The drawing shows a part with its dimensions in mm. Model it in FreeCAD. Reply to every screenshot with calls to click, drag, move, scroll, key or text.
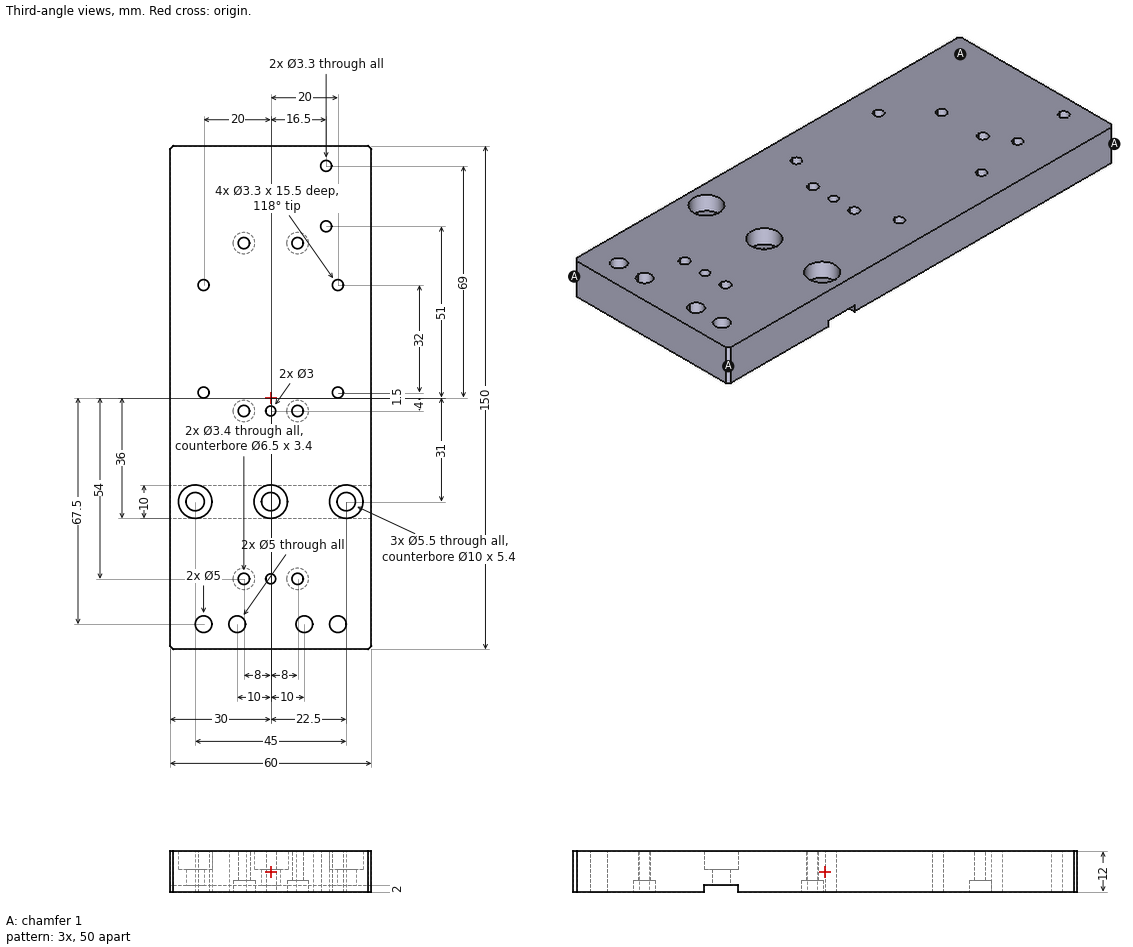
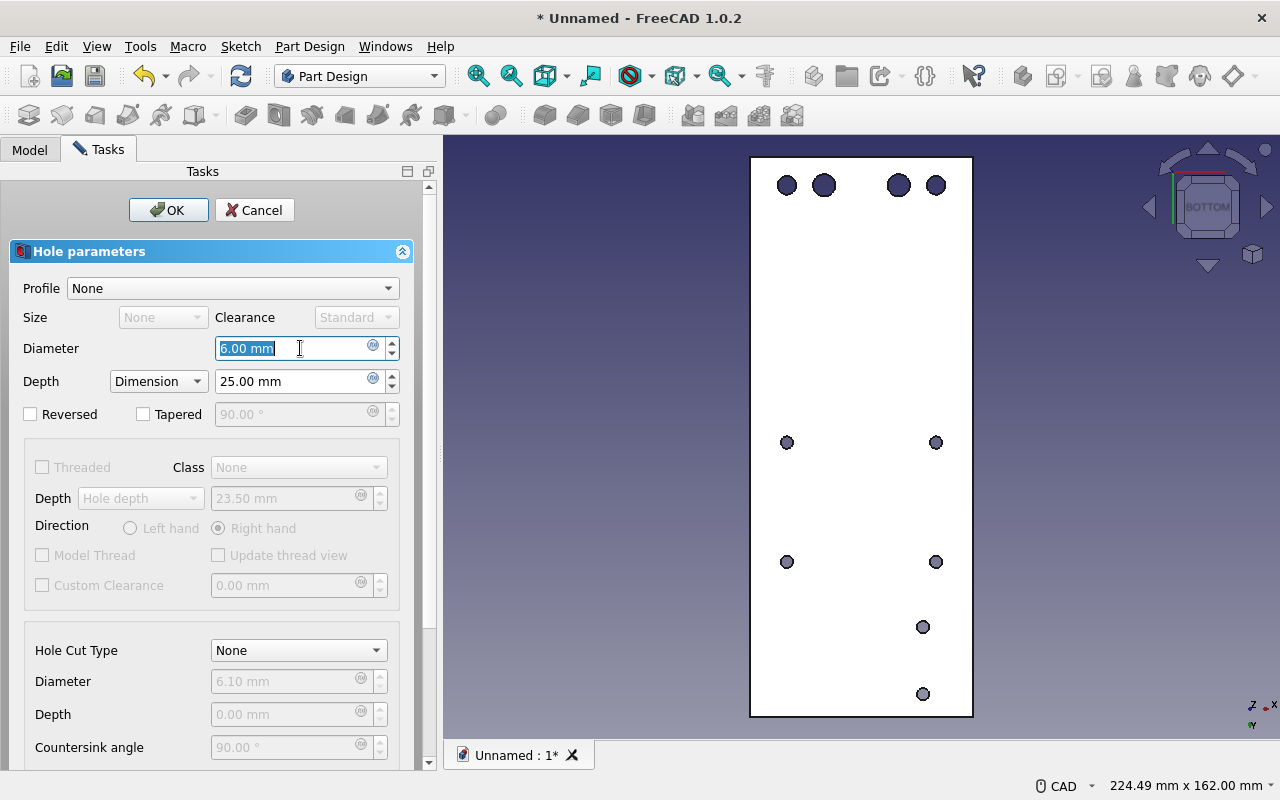
text(5)
key(Tab)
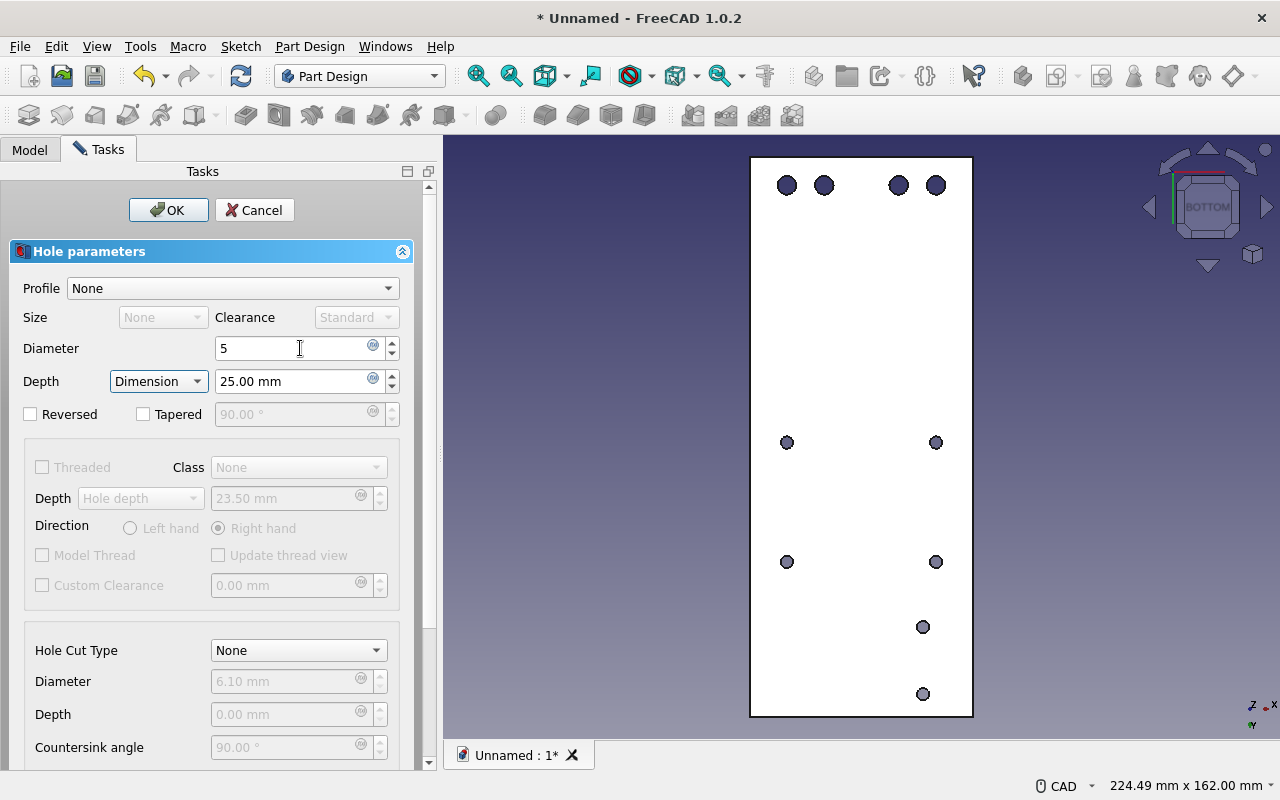
click(160, 382)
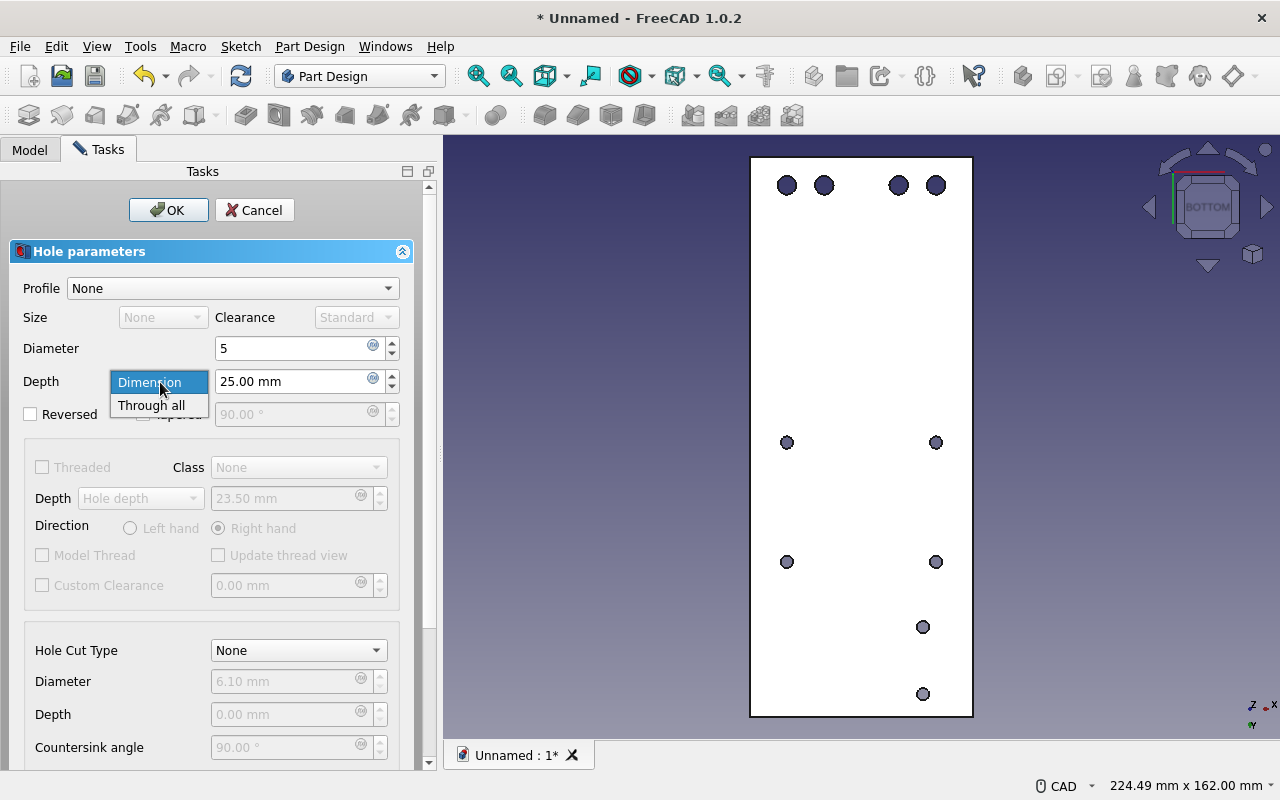
click(158, 406)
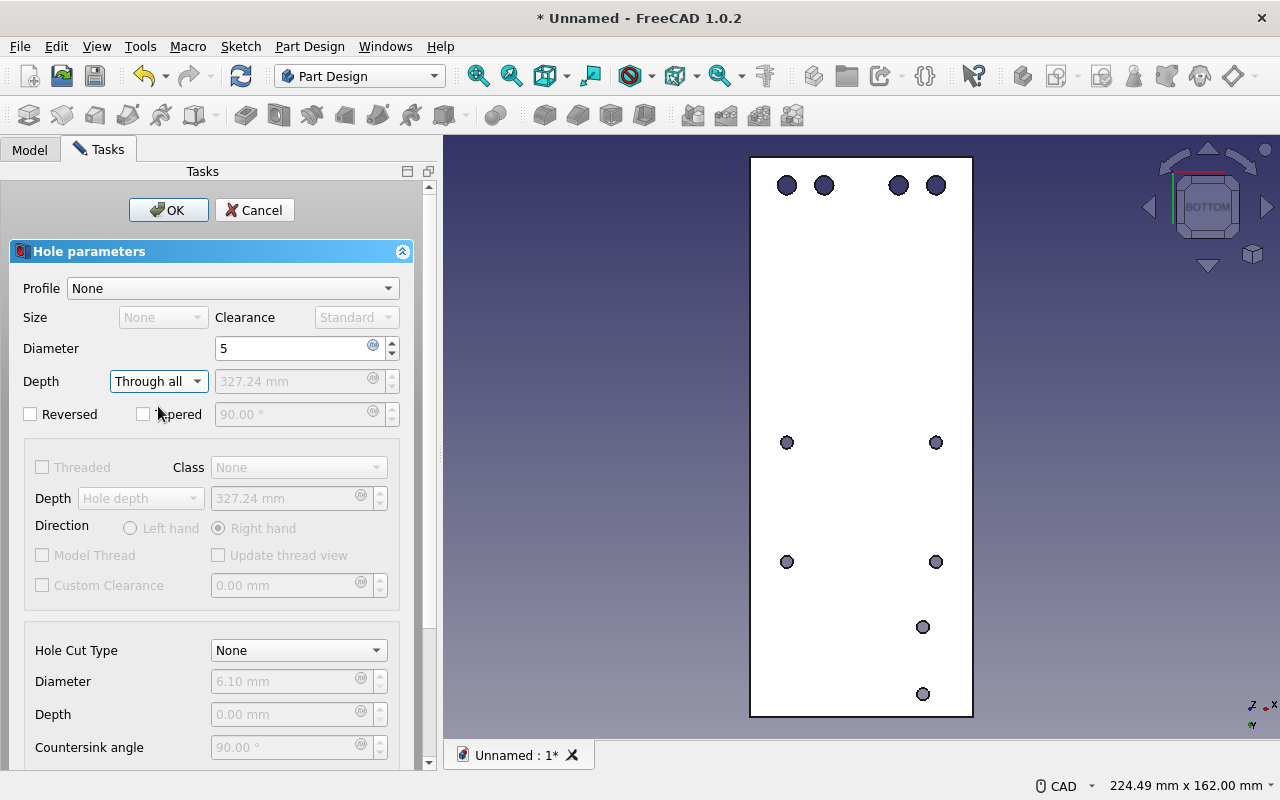
click(169, 210)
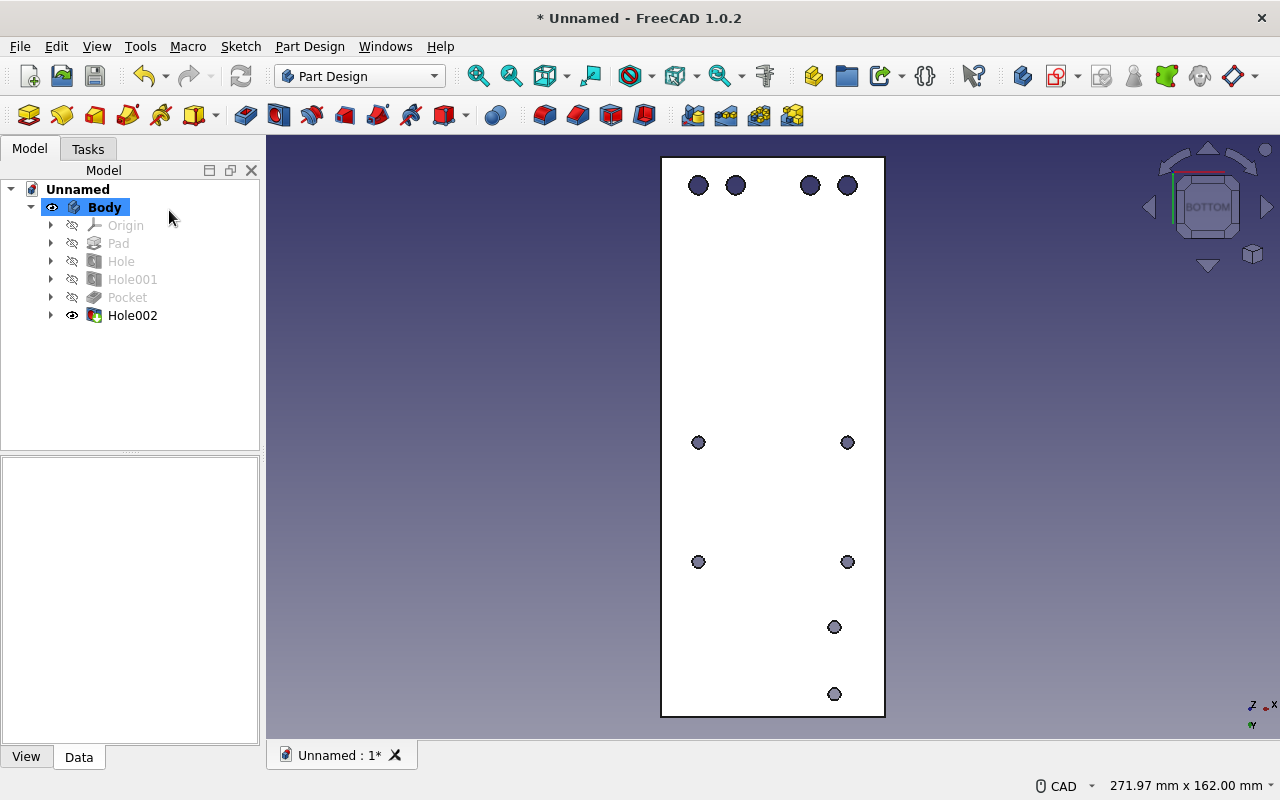
key(0)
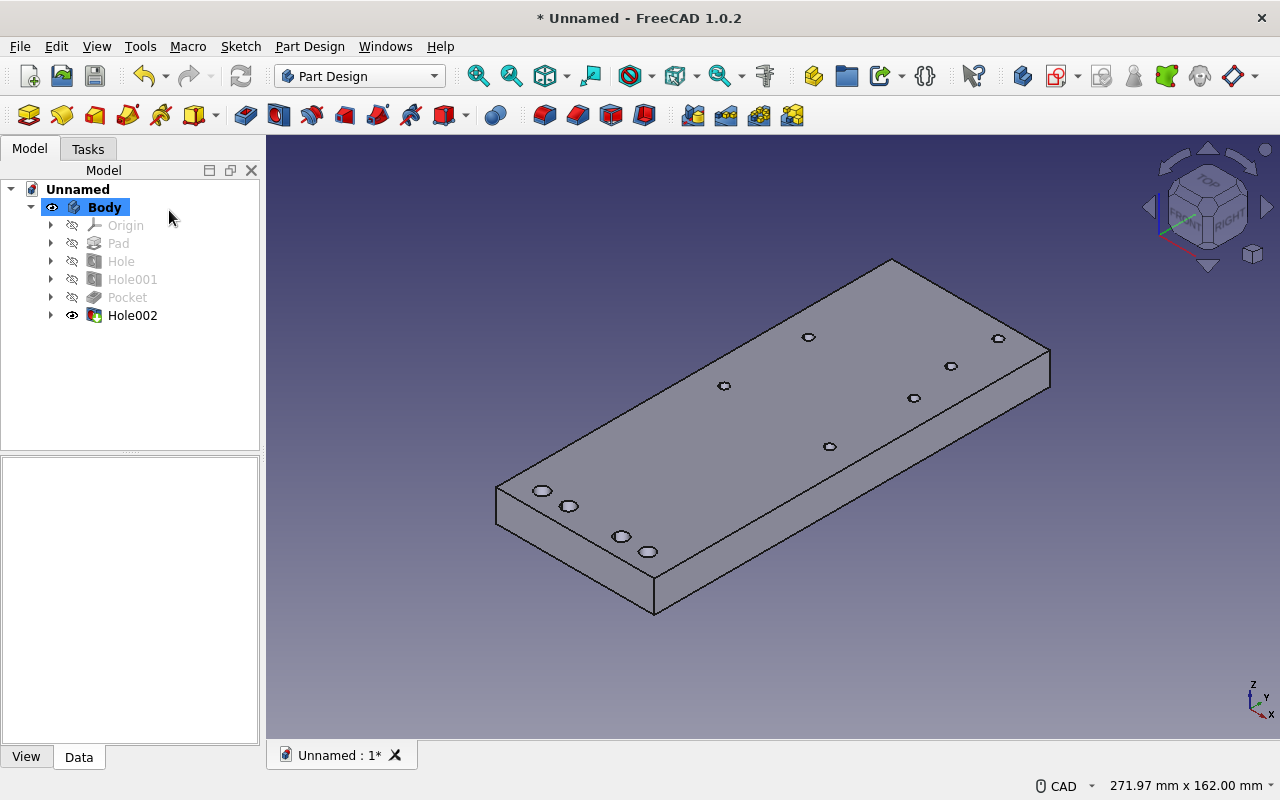
click(654, 596)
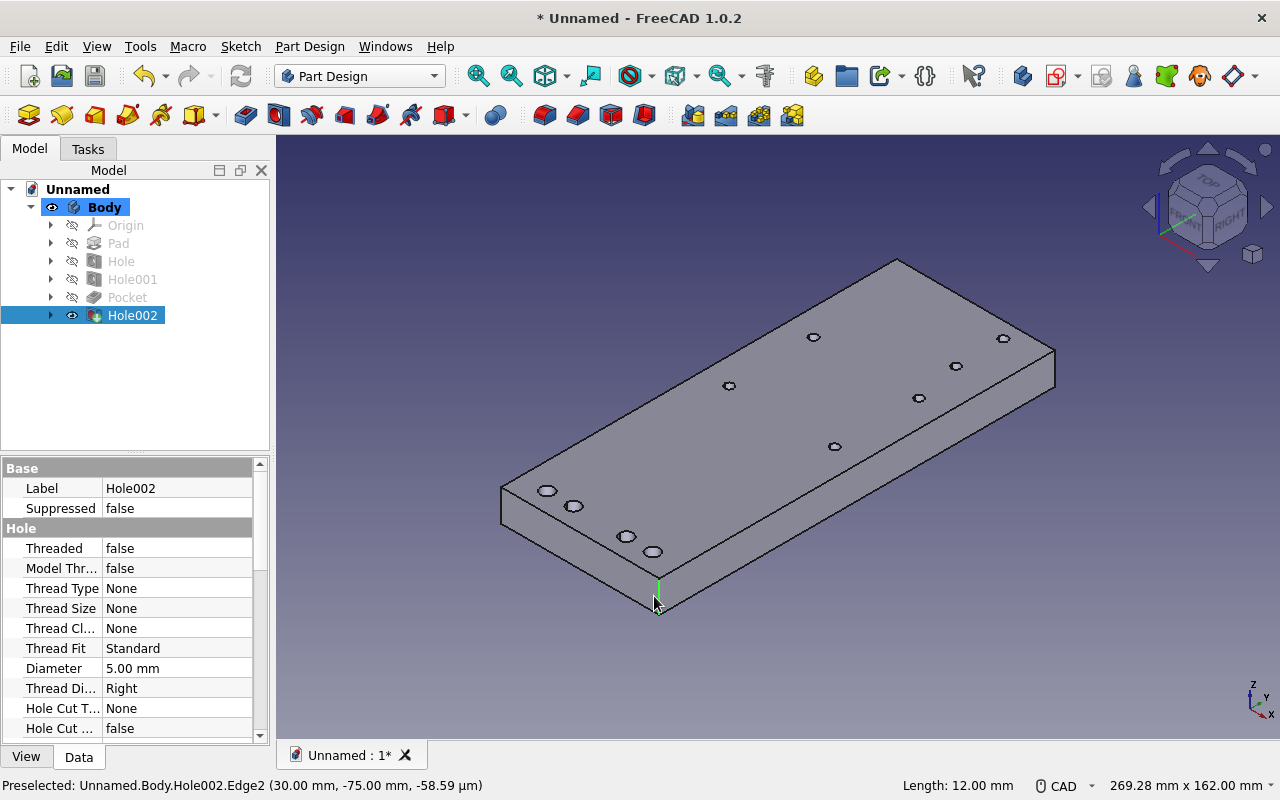
key(2)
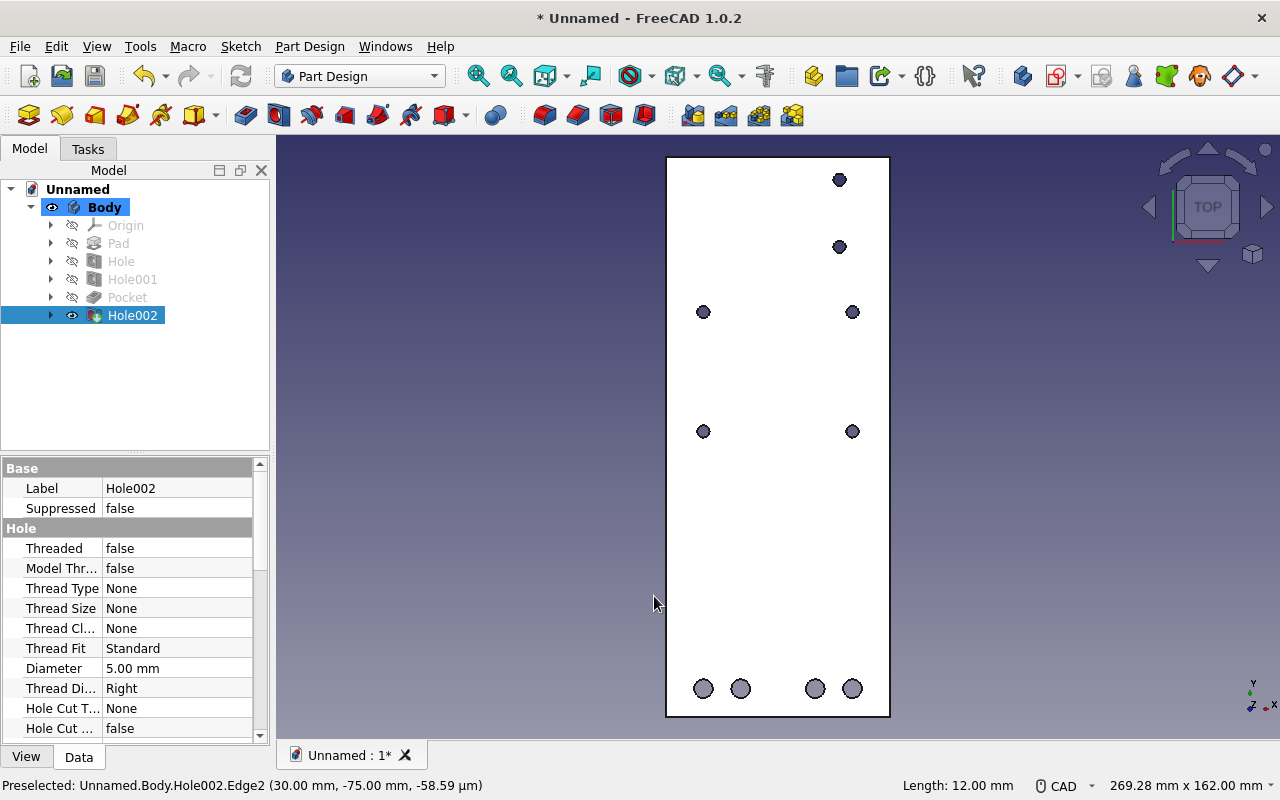
key(1)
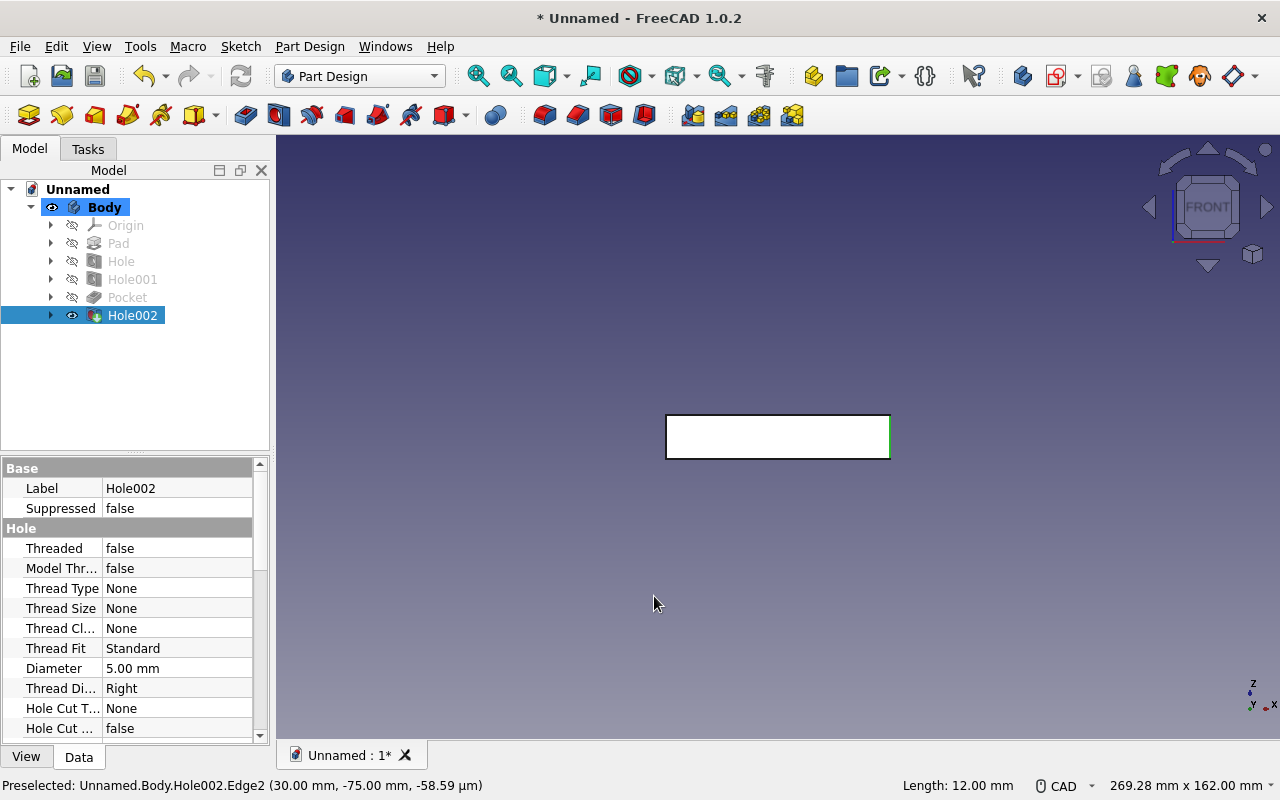
click(479, 76)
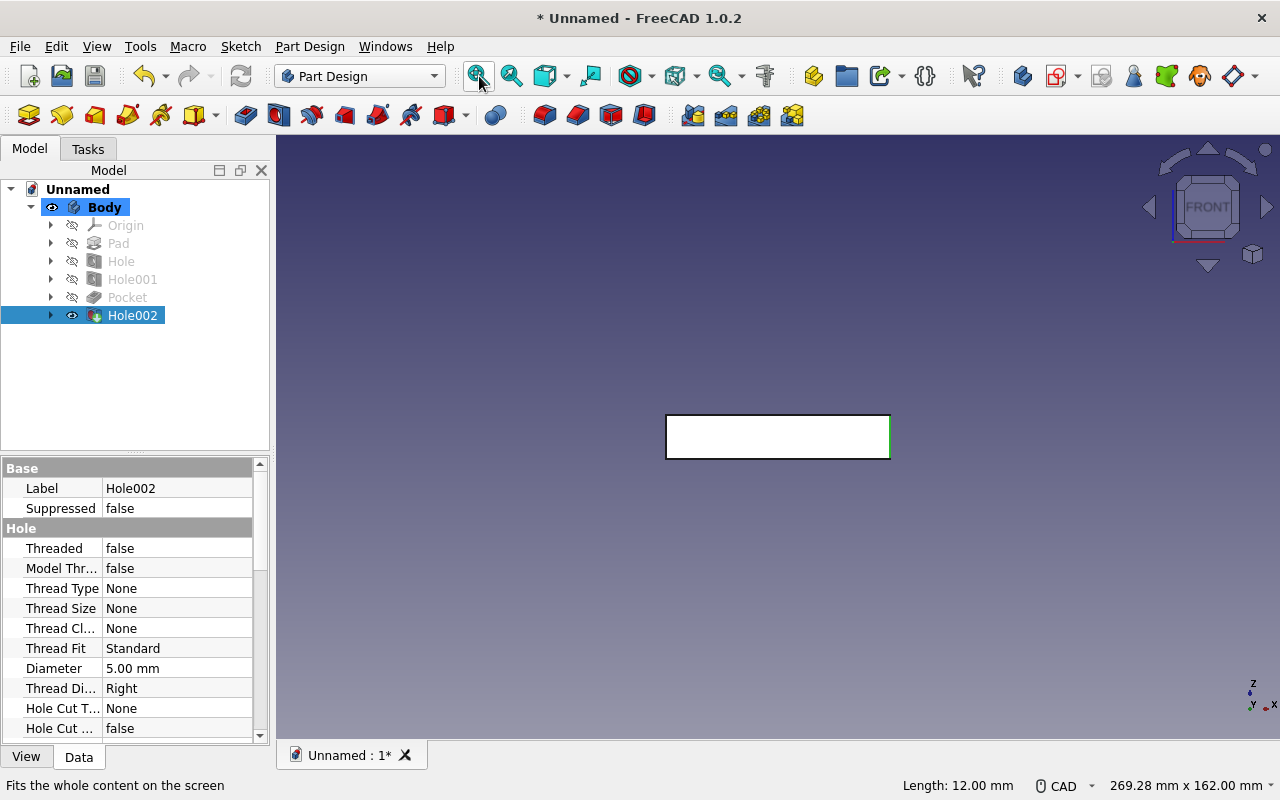
click(666, 436, ctrl)